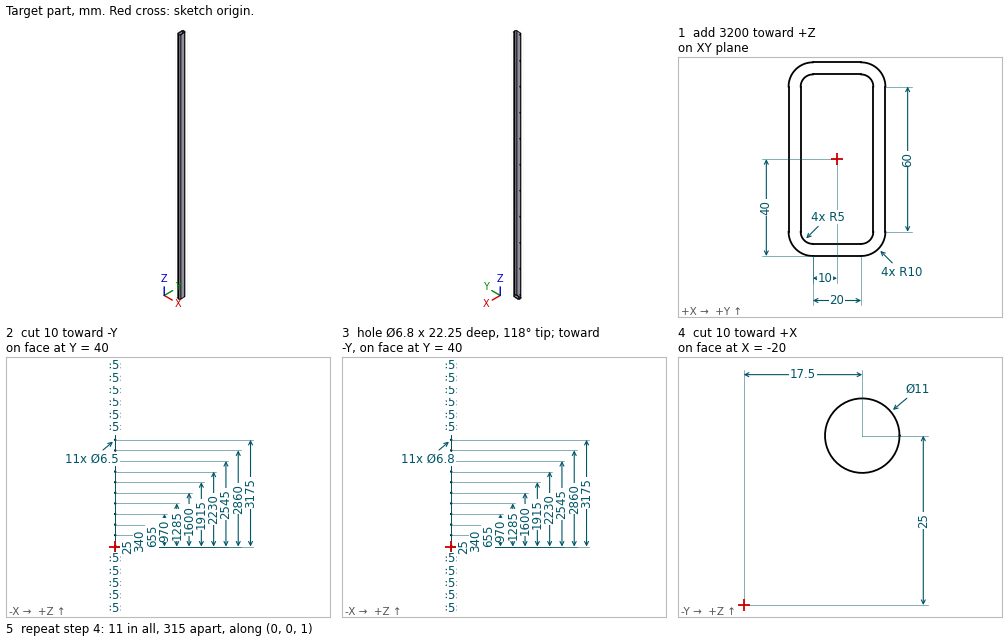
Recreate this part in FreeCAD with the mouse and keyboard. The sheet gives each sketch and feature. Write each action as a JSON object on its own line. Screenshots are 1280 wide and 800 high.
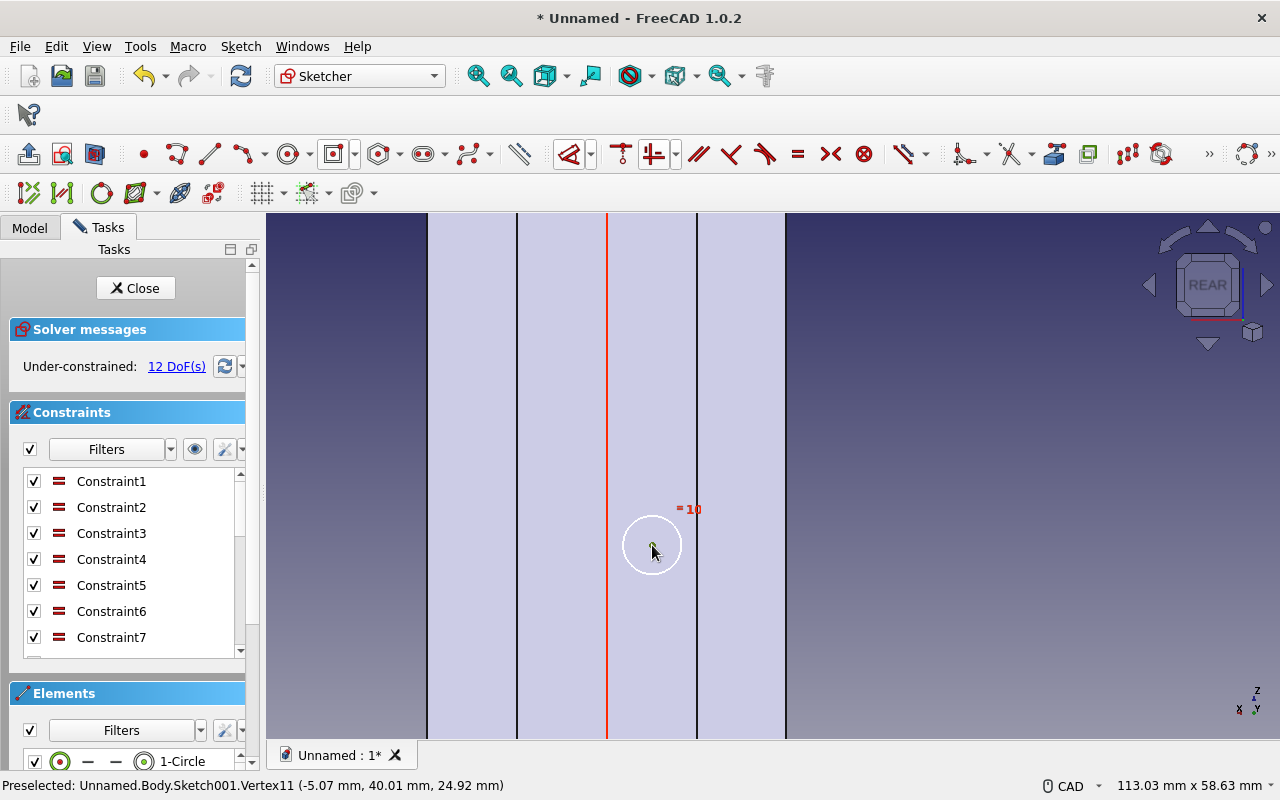
{"action": "left_click", "coordinate": [590, 154]}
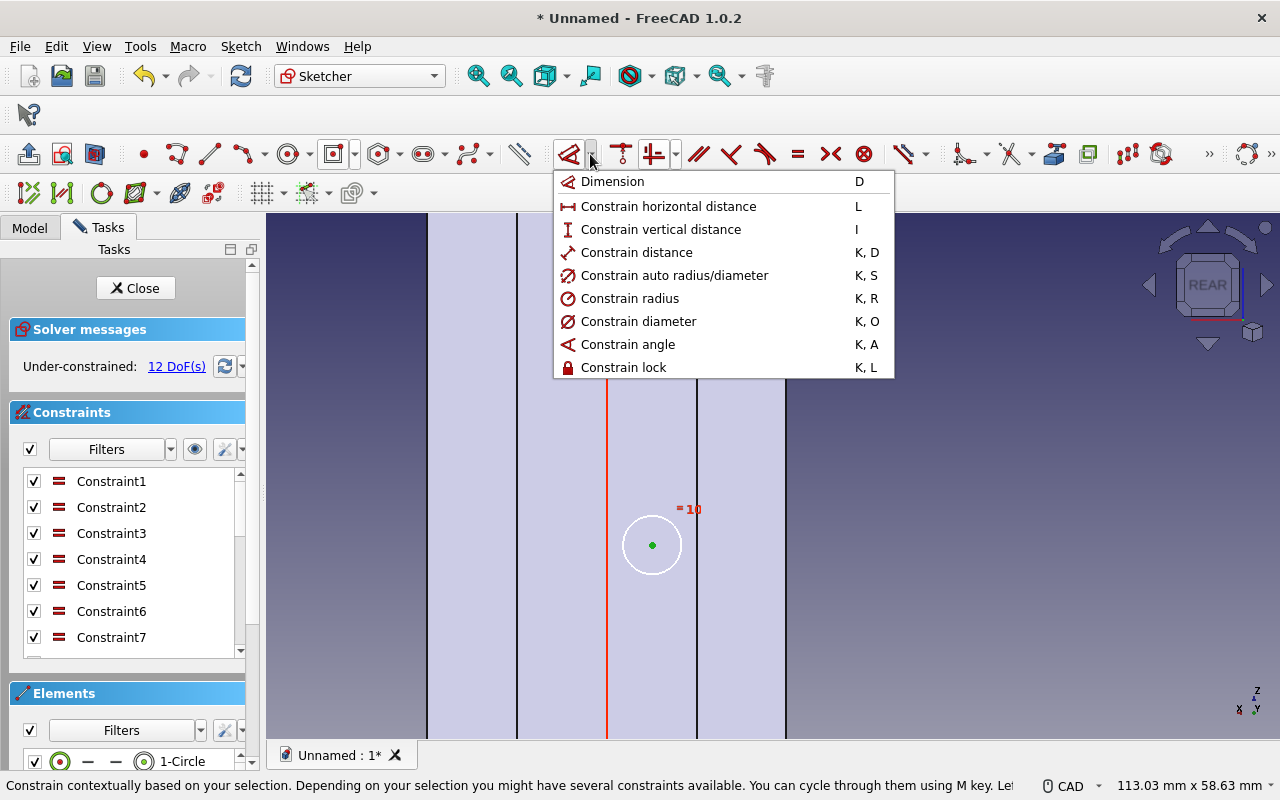
{"action": "left_click", "coordinate": [724, 206]}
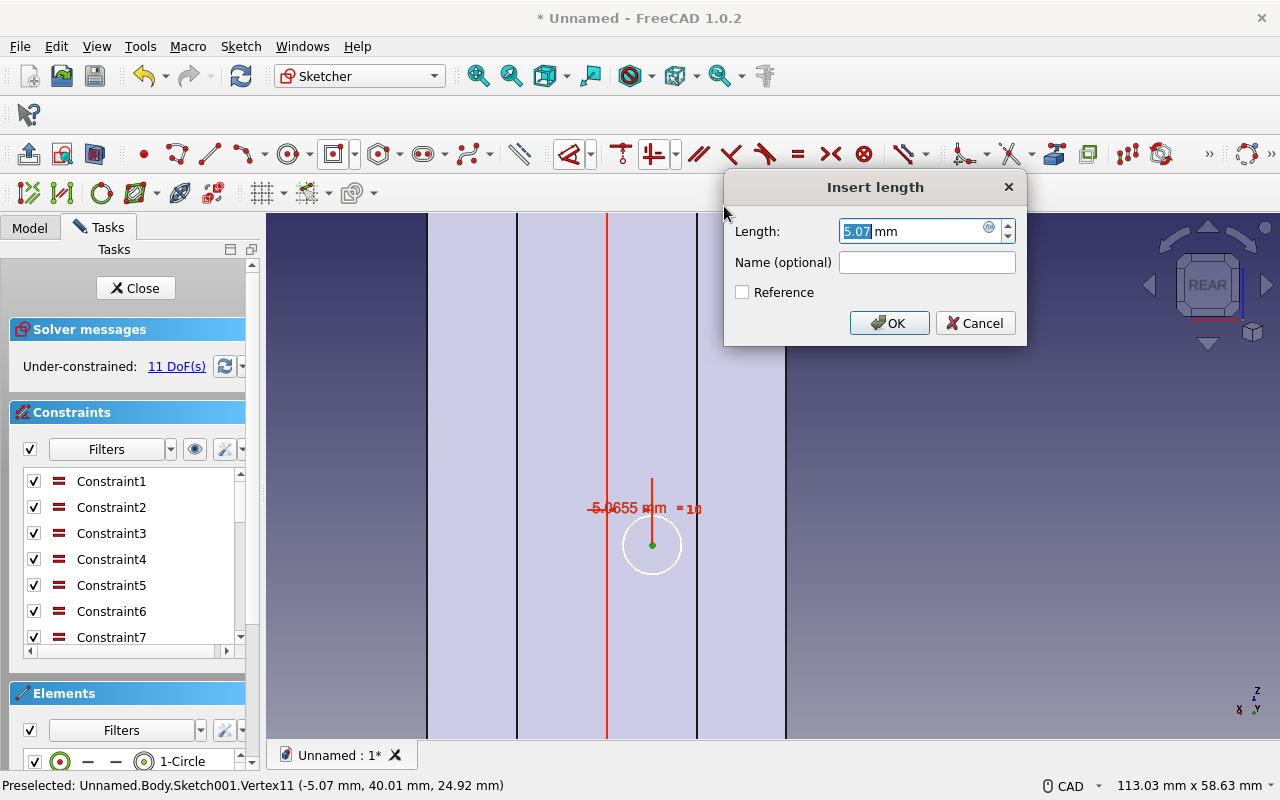
{"action": "type", "text": "5"}
{"action": "key", "text": "Return"}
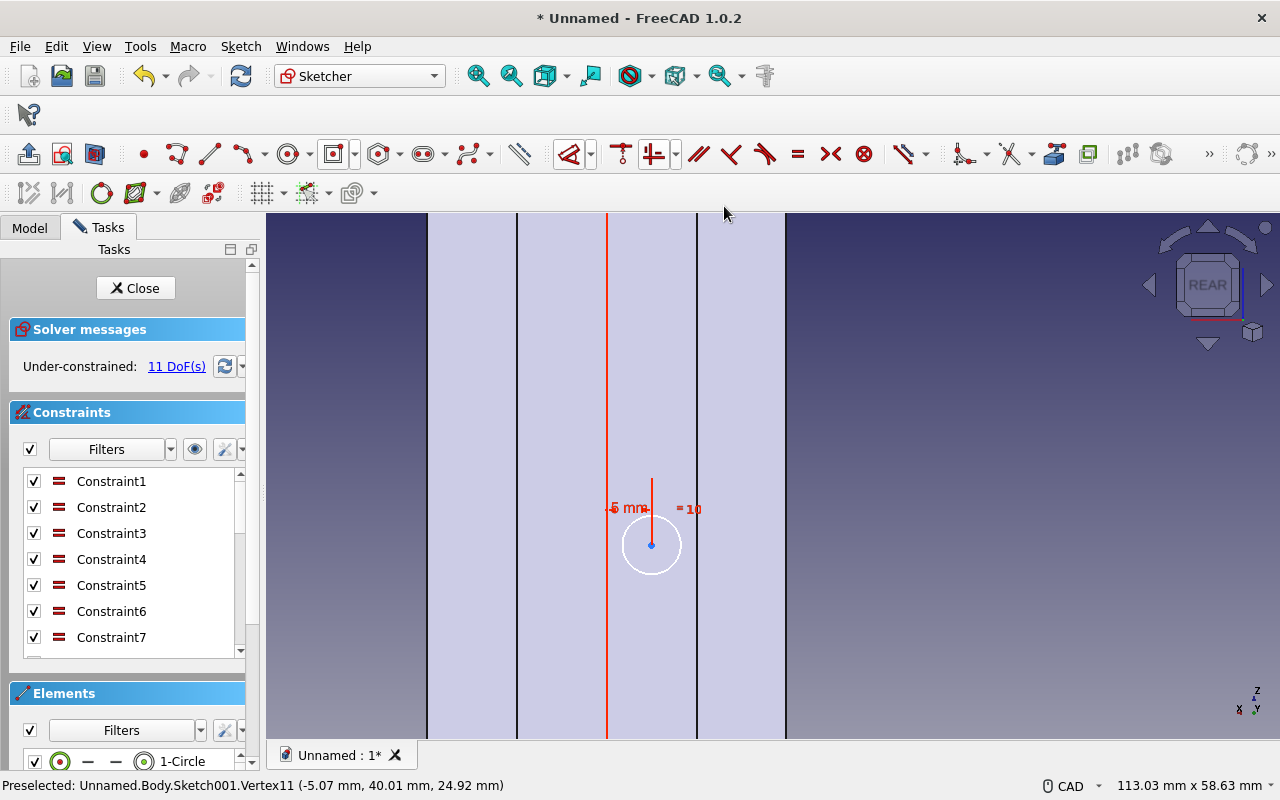
{"action": "scroll", "coordinate": [704, 476], "scroll_direction": "down", "scroll_amount": 15}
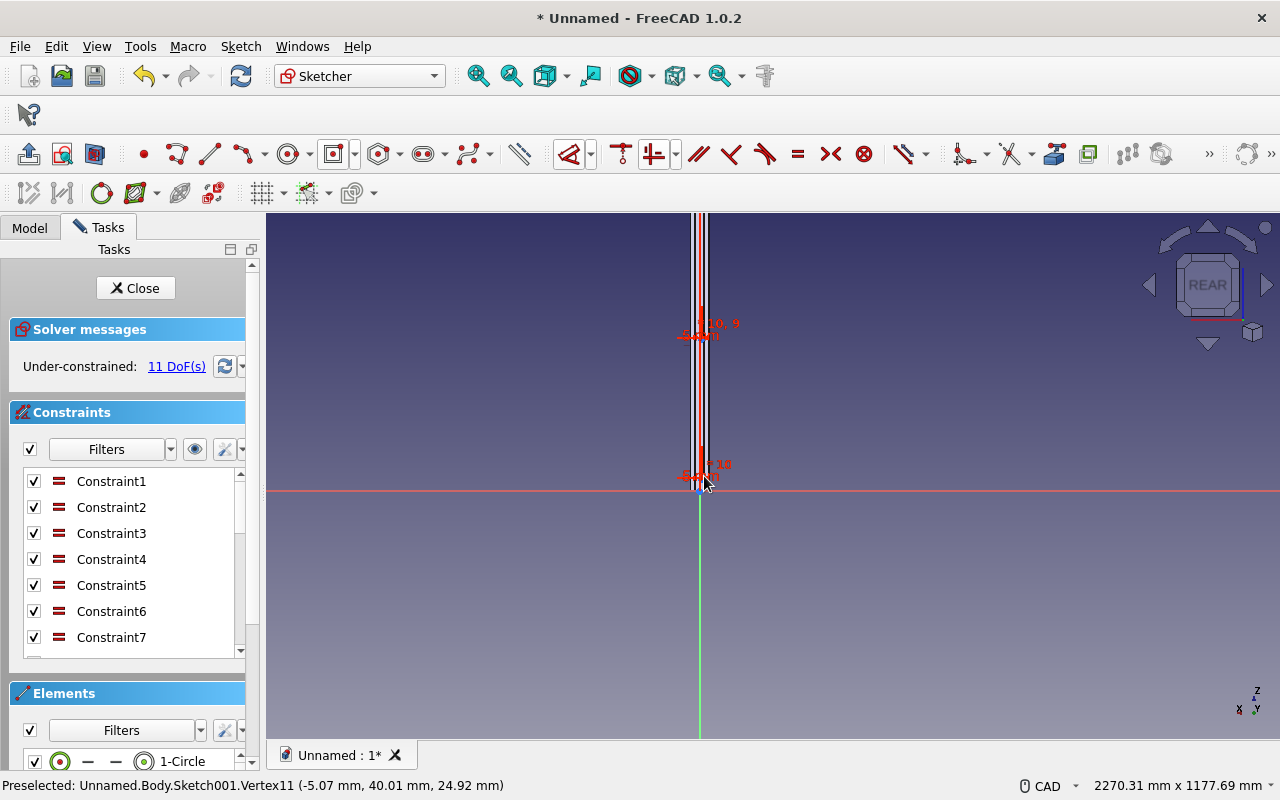
{"action": "scroll", "coordinate": [706, 703], "scroll_direction": "down", "scroll_amount": 7}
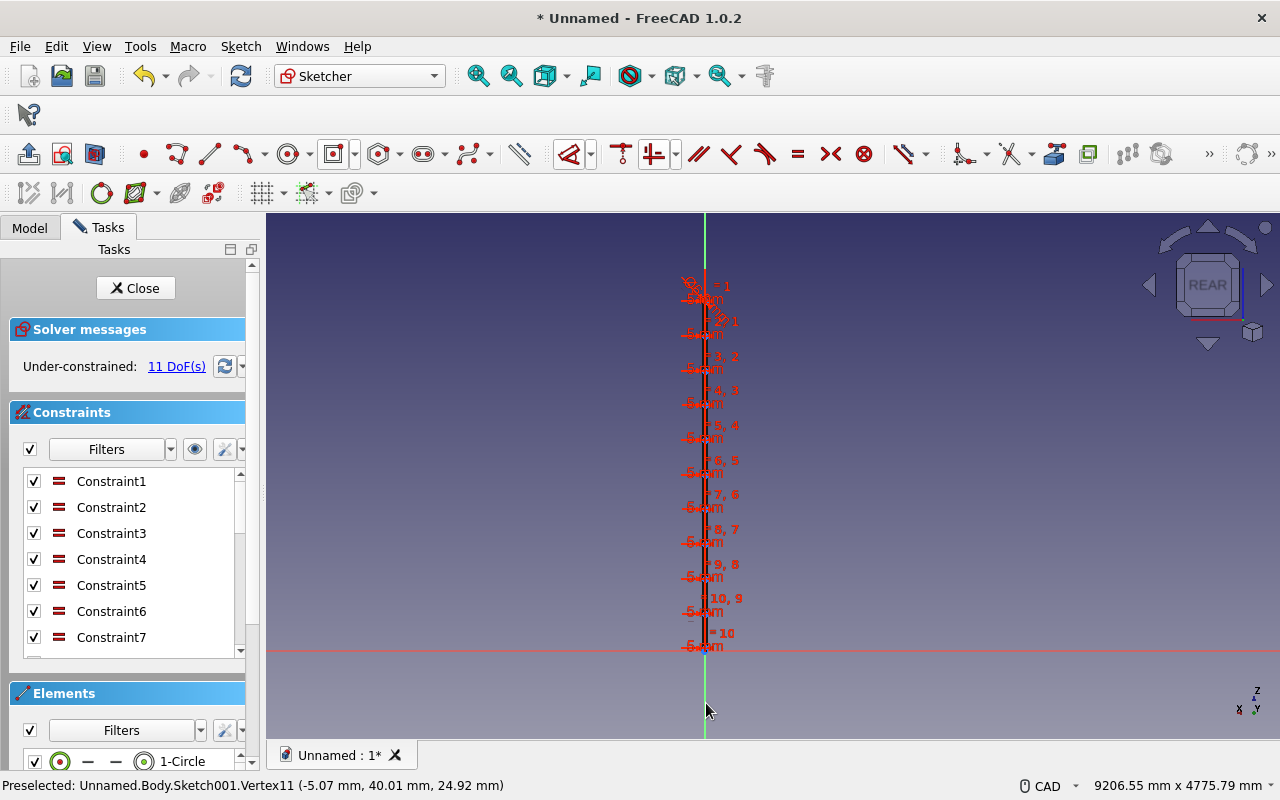
{"action": "scroll", "coordinate": [705, 649], "scroll_direction": "up", "scroll_amount": 14}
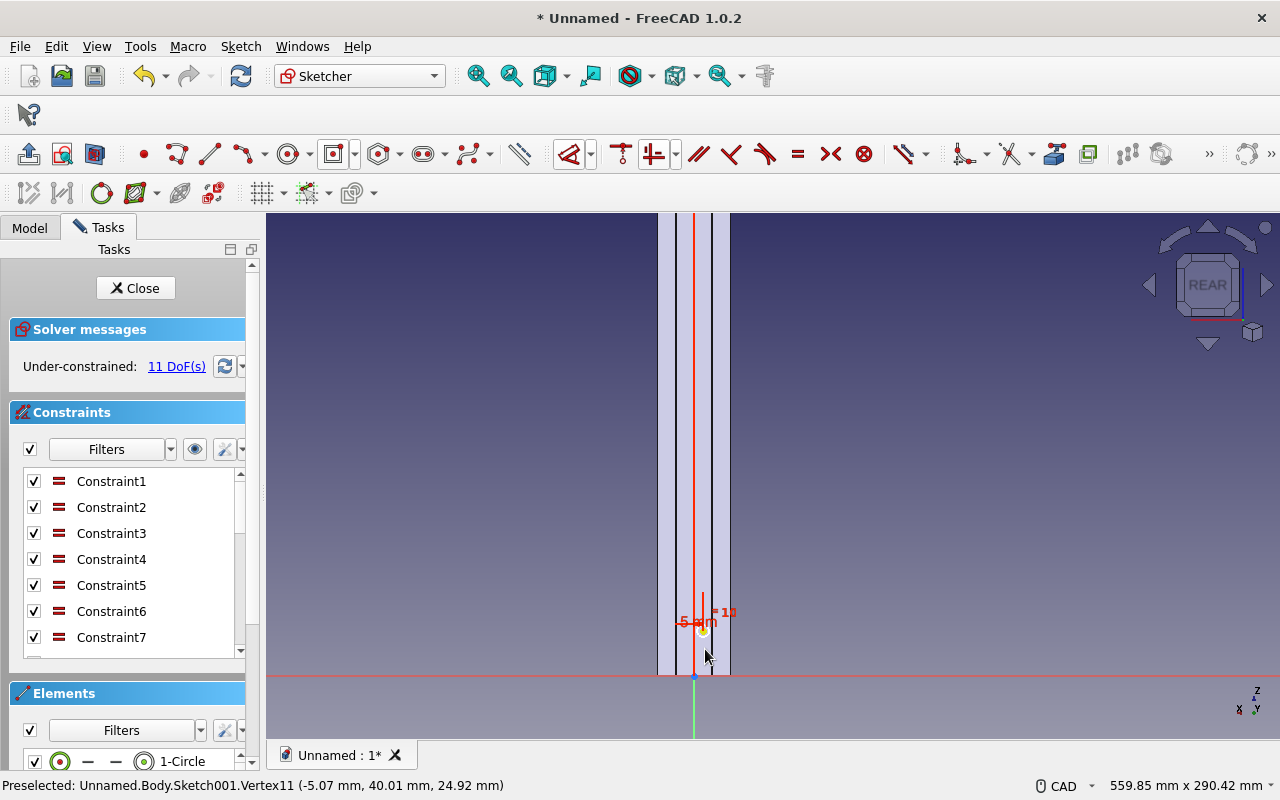
{"action": "left_click", "coordinate": [703, 631]}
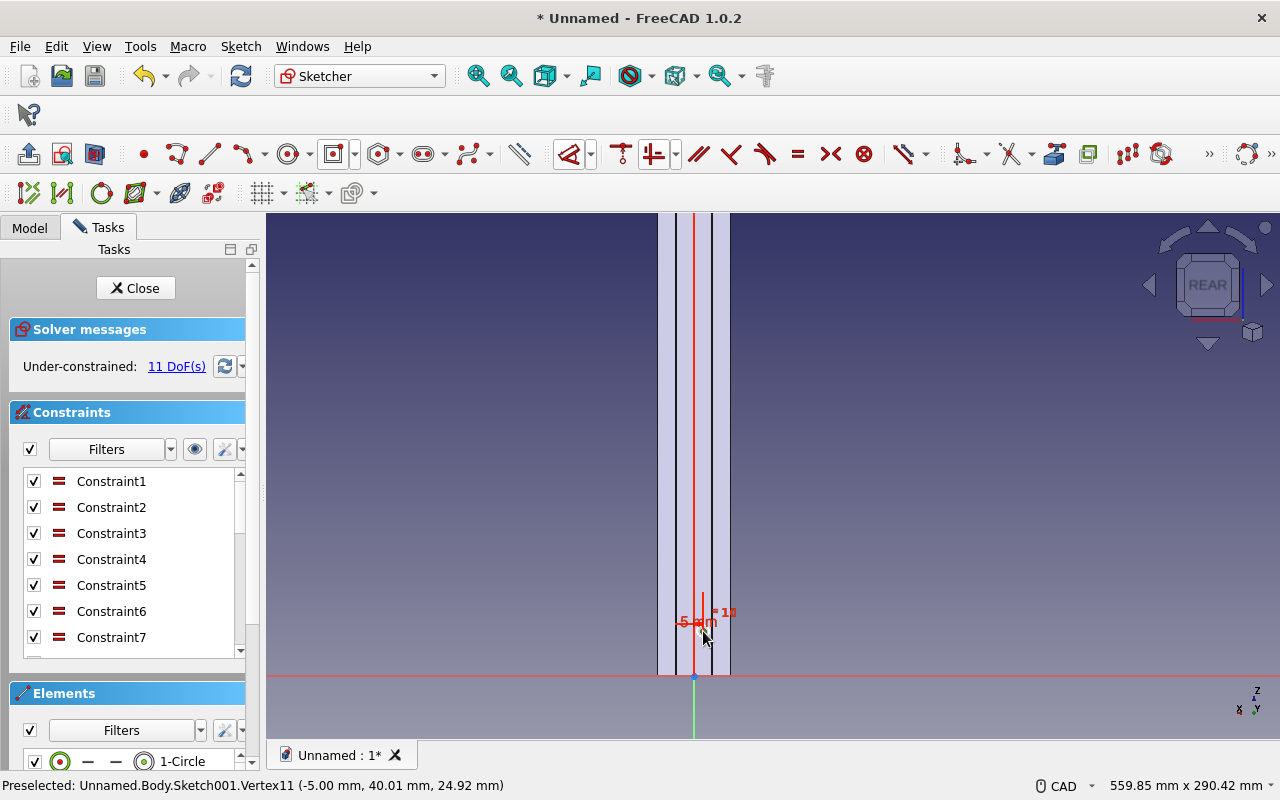
{"action": "key", "text": "i"}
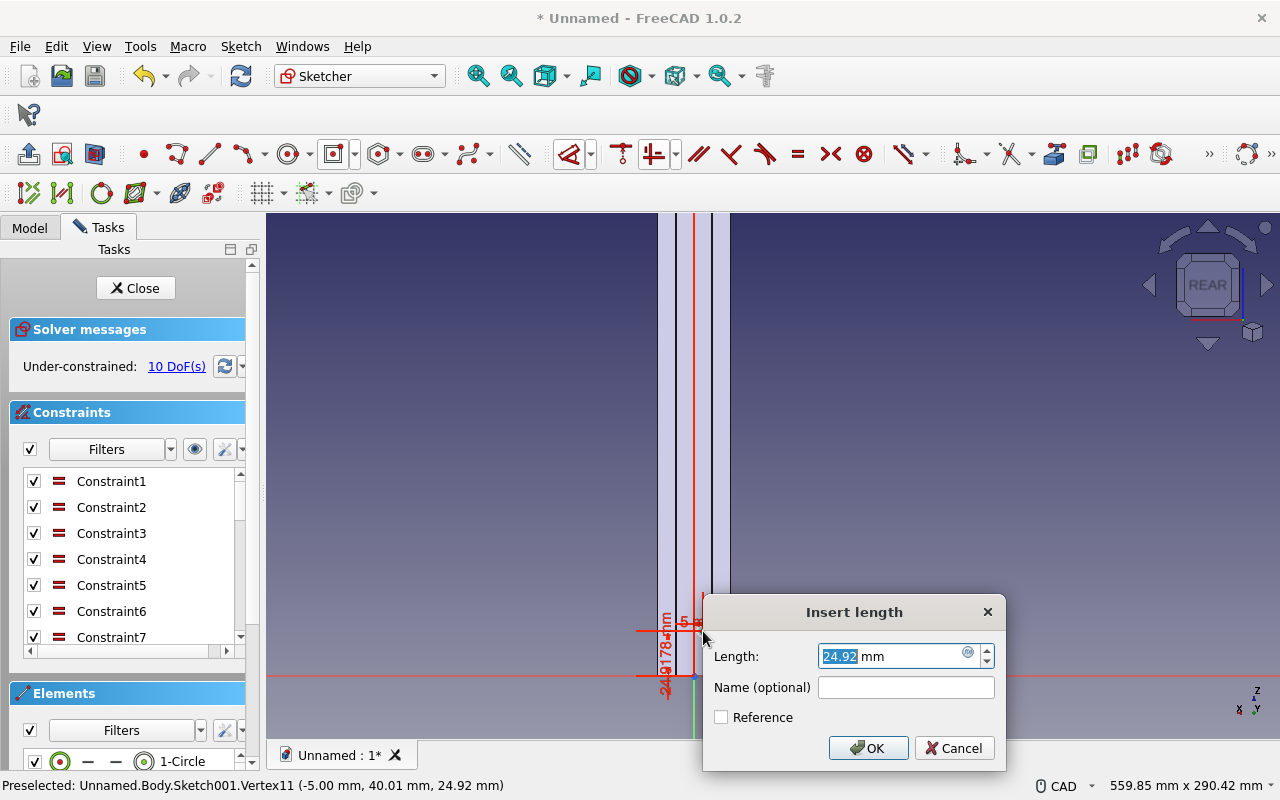
{"action": "type", "text": "25"}
{"action": "key", "text": "Return"}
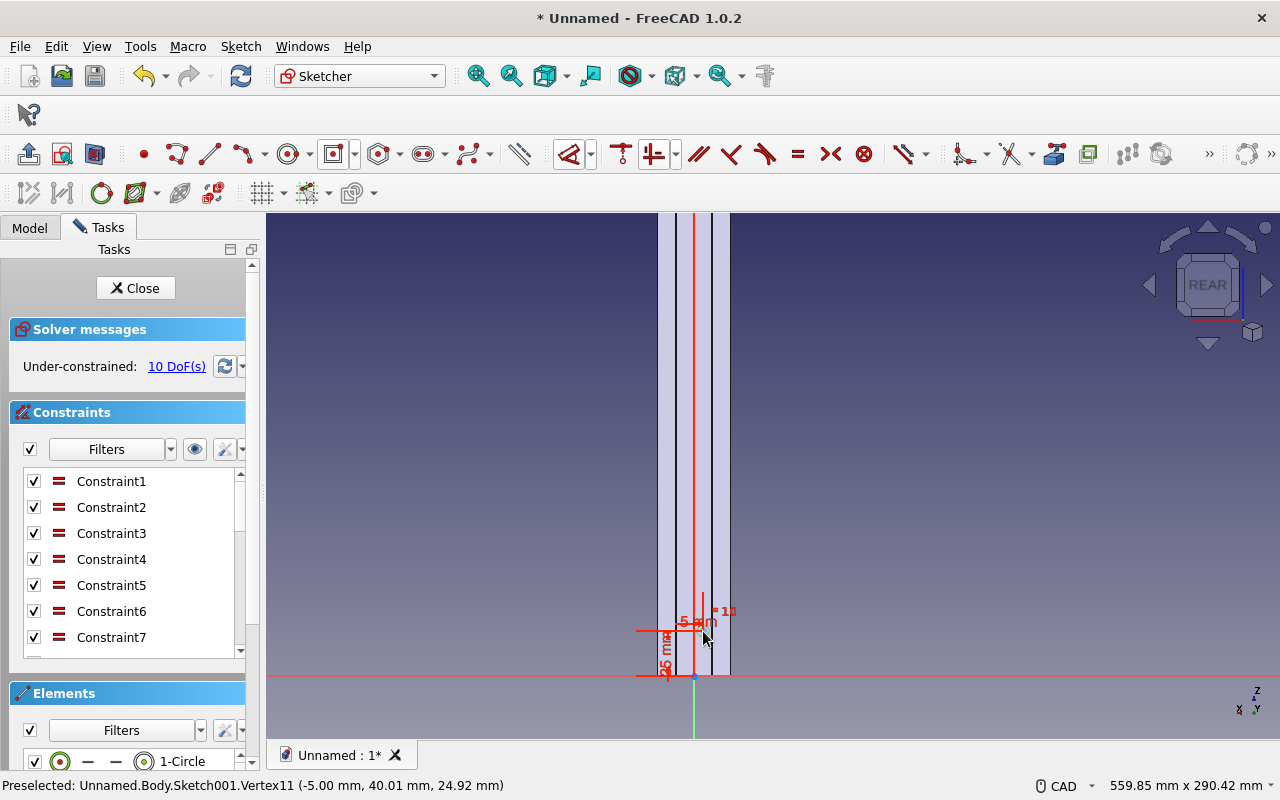
{"action": "scroll", "coordinate": [705, 649], "scroll_direction": "down", "scroll_amount": 14}